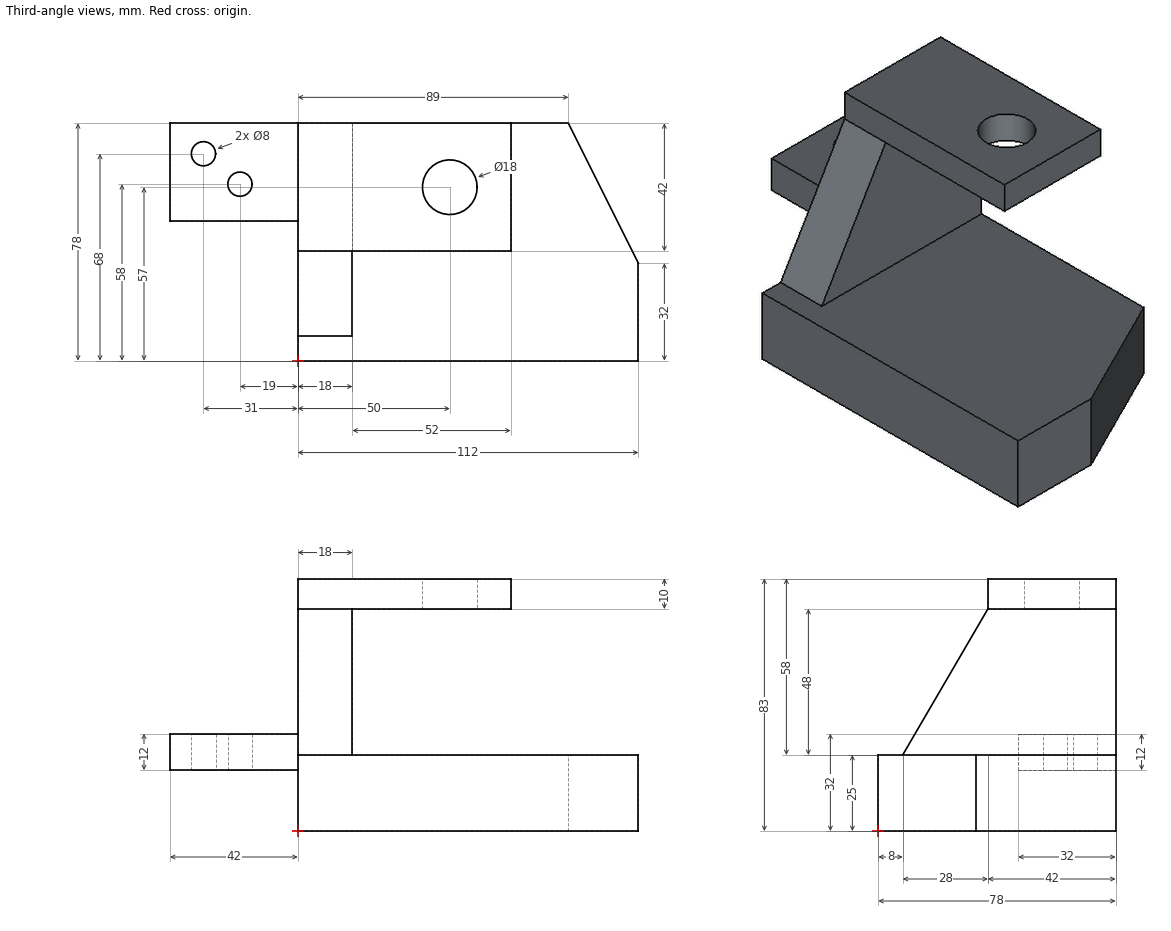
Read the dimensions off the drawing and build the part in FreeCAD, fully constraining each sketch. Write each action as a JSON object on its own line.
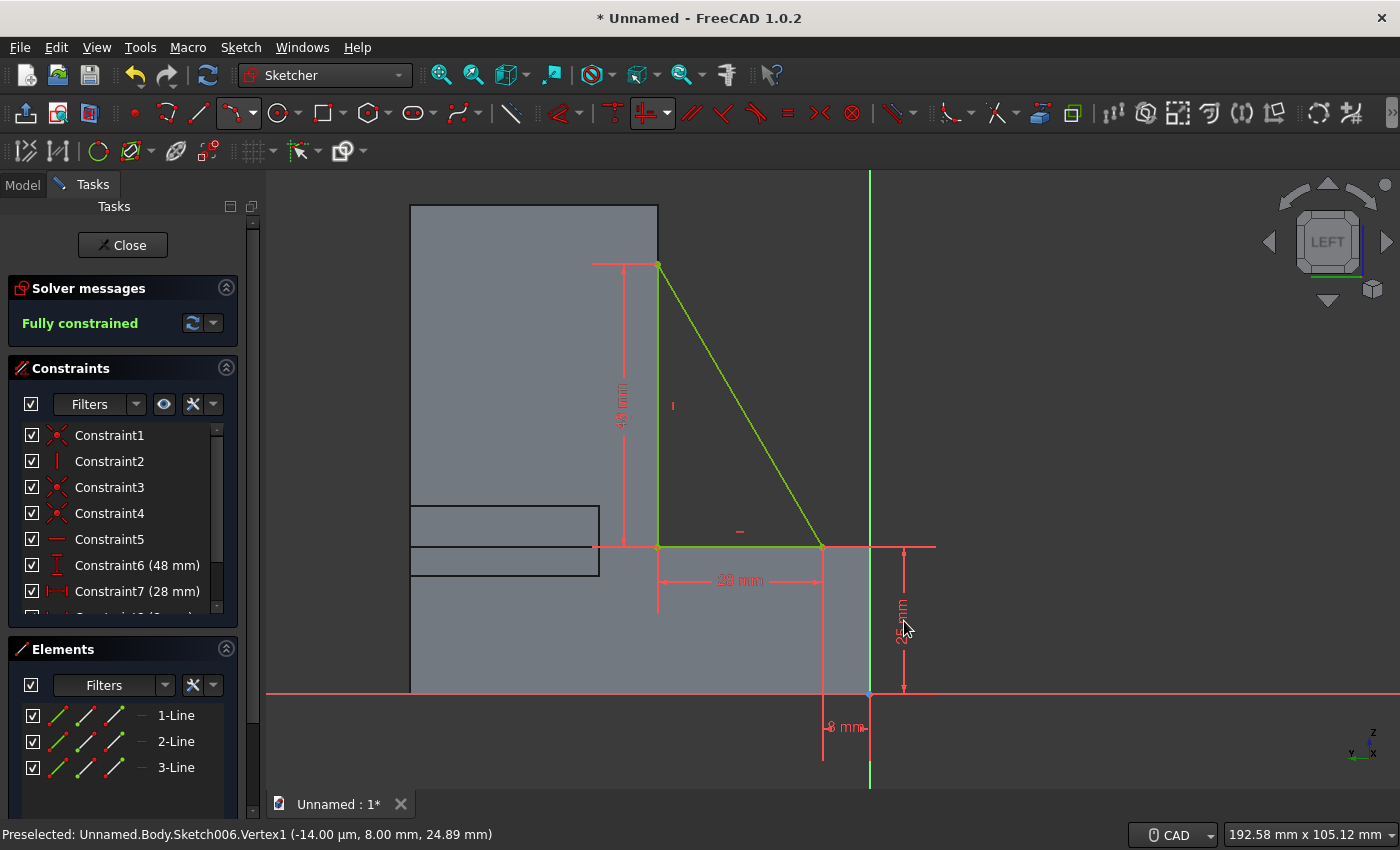
{"action": "left_click", "coordinate": [123, 245]}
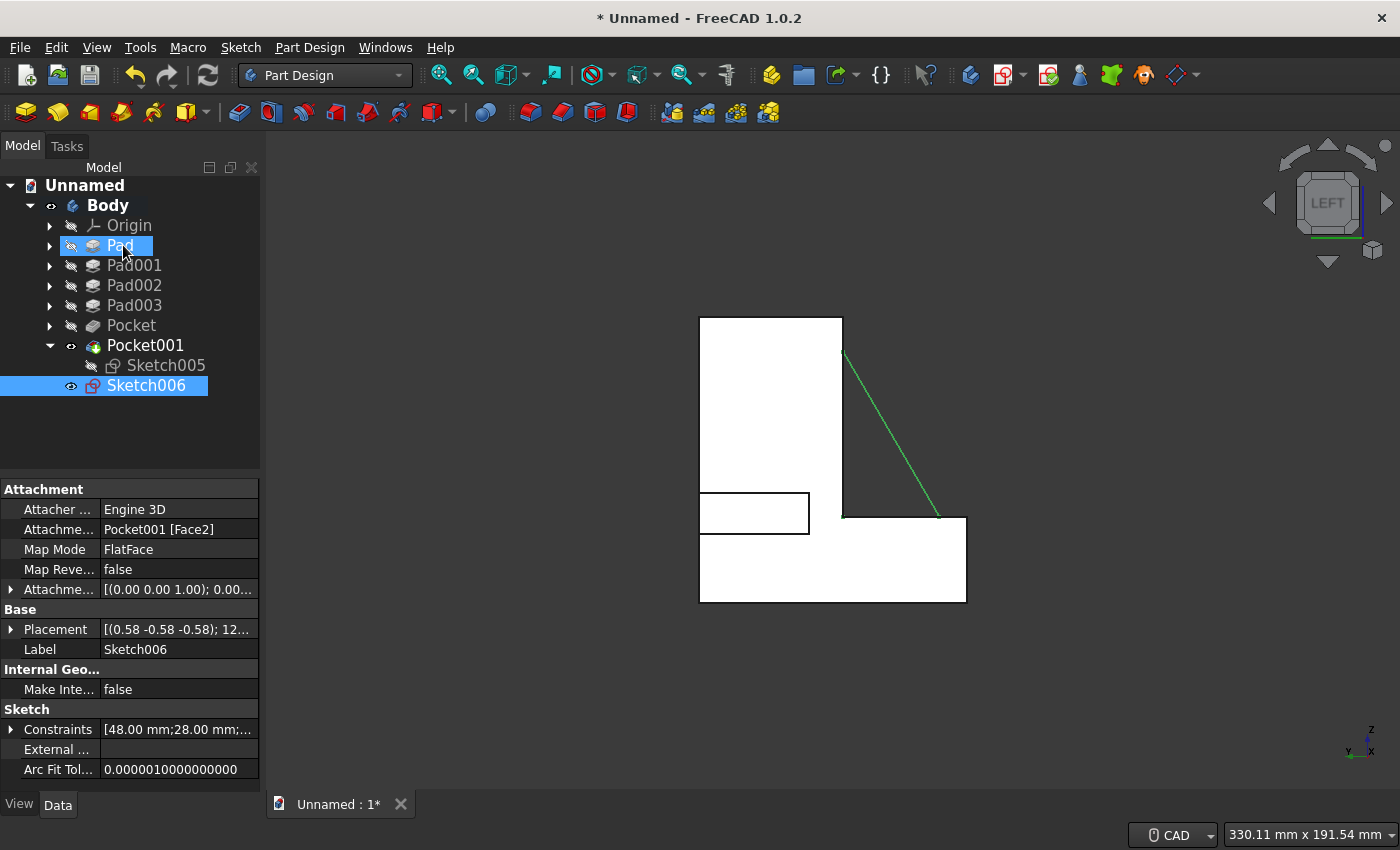
{"action": "left_click", "coordinate": [26, 112]}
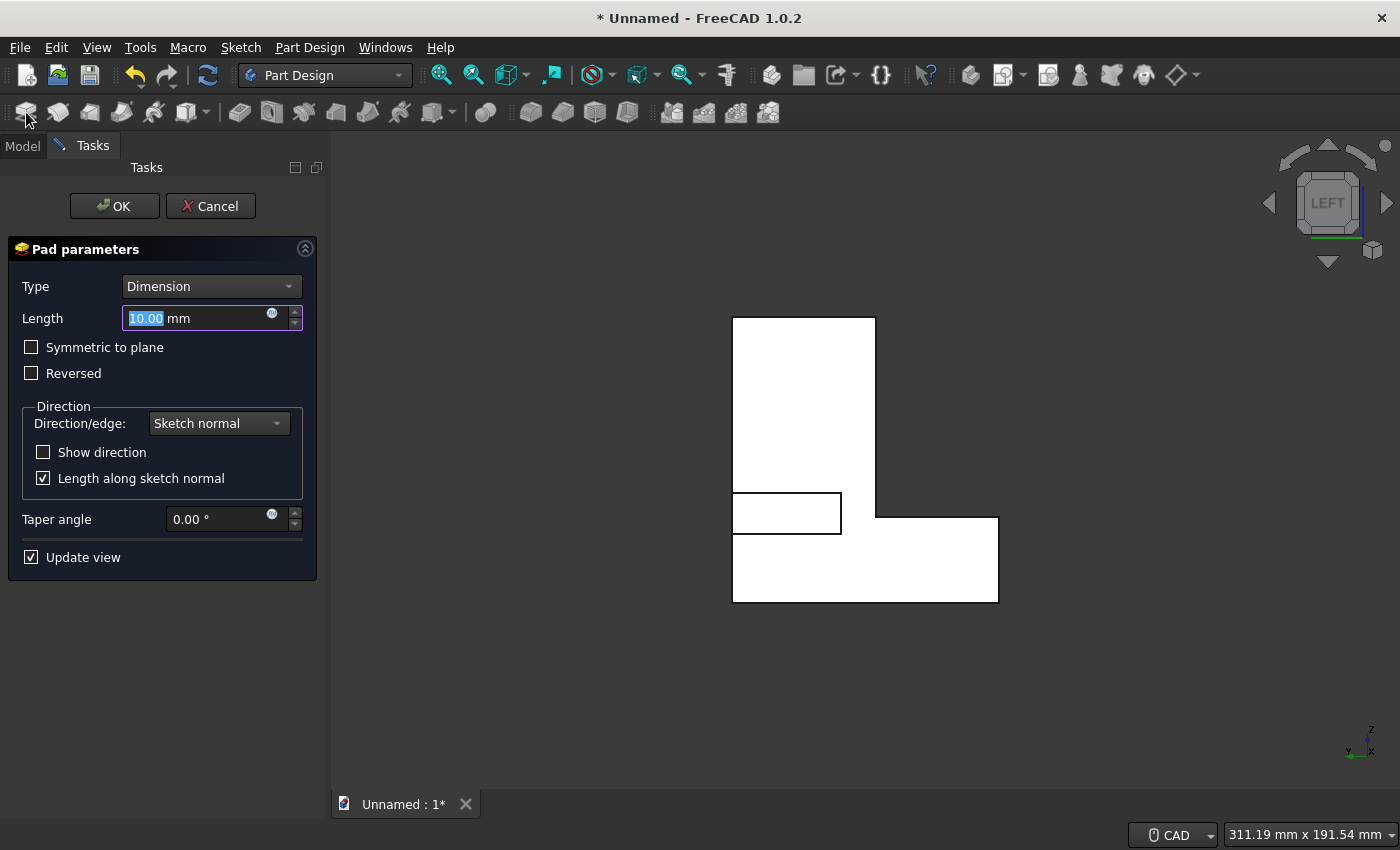
{"action": "type", "text": "18"}
{"action": "key", "text": "Tab"}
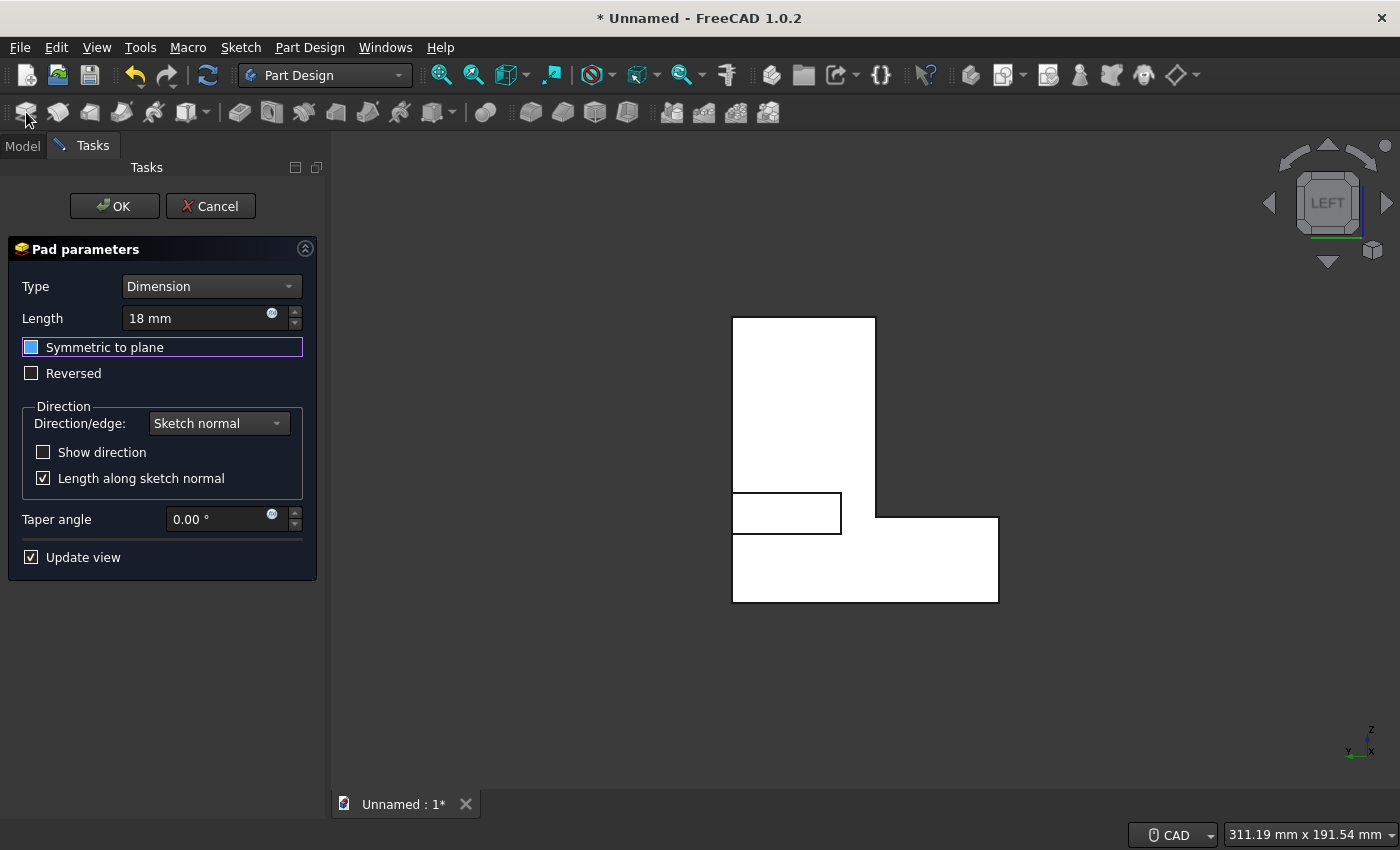
{"action": "left_click", "coordinate": [30, 373]}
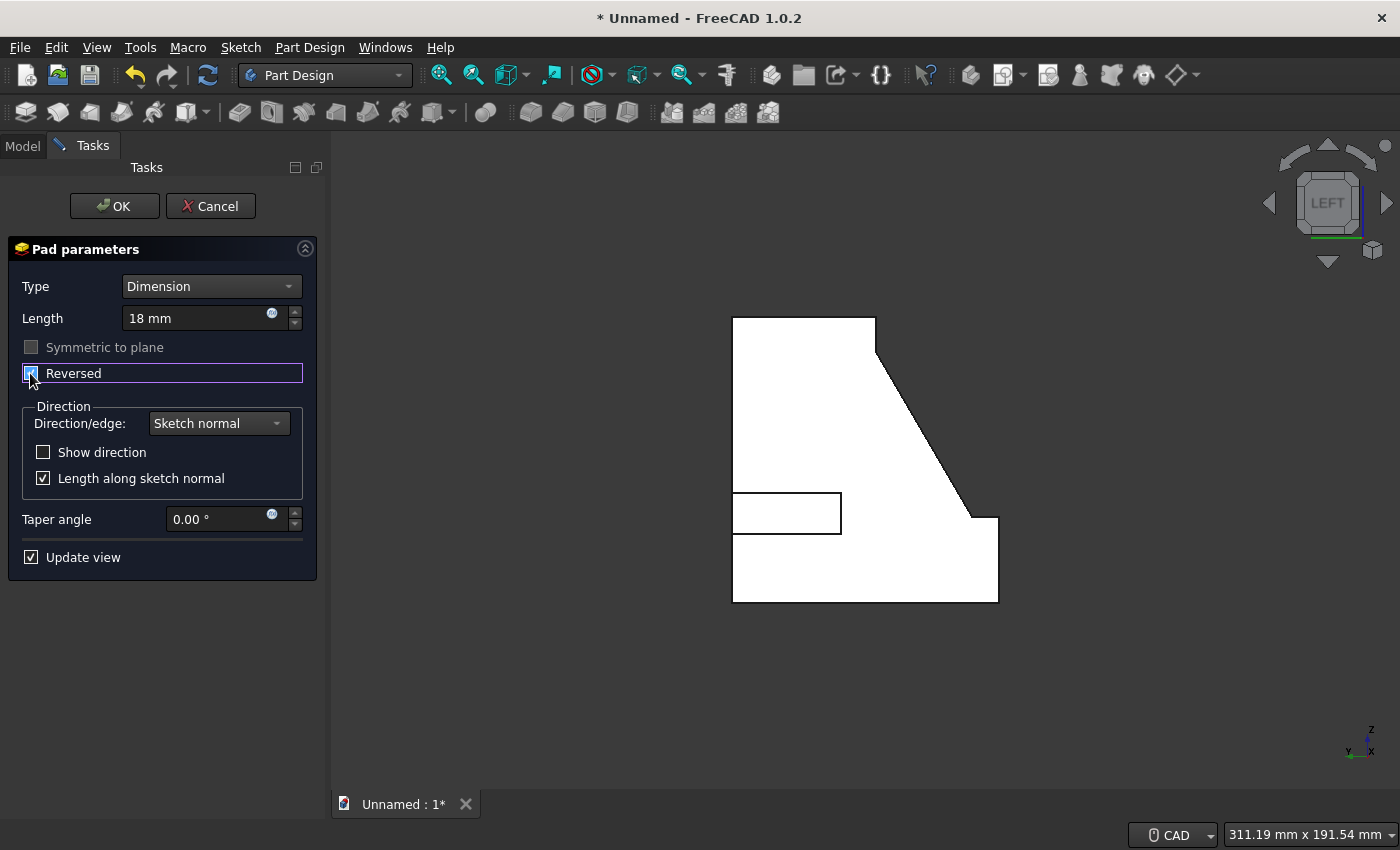
{"action": "left_click", "coordinate": [115, 206]}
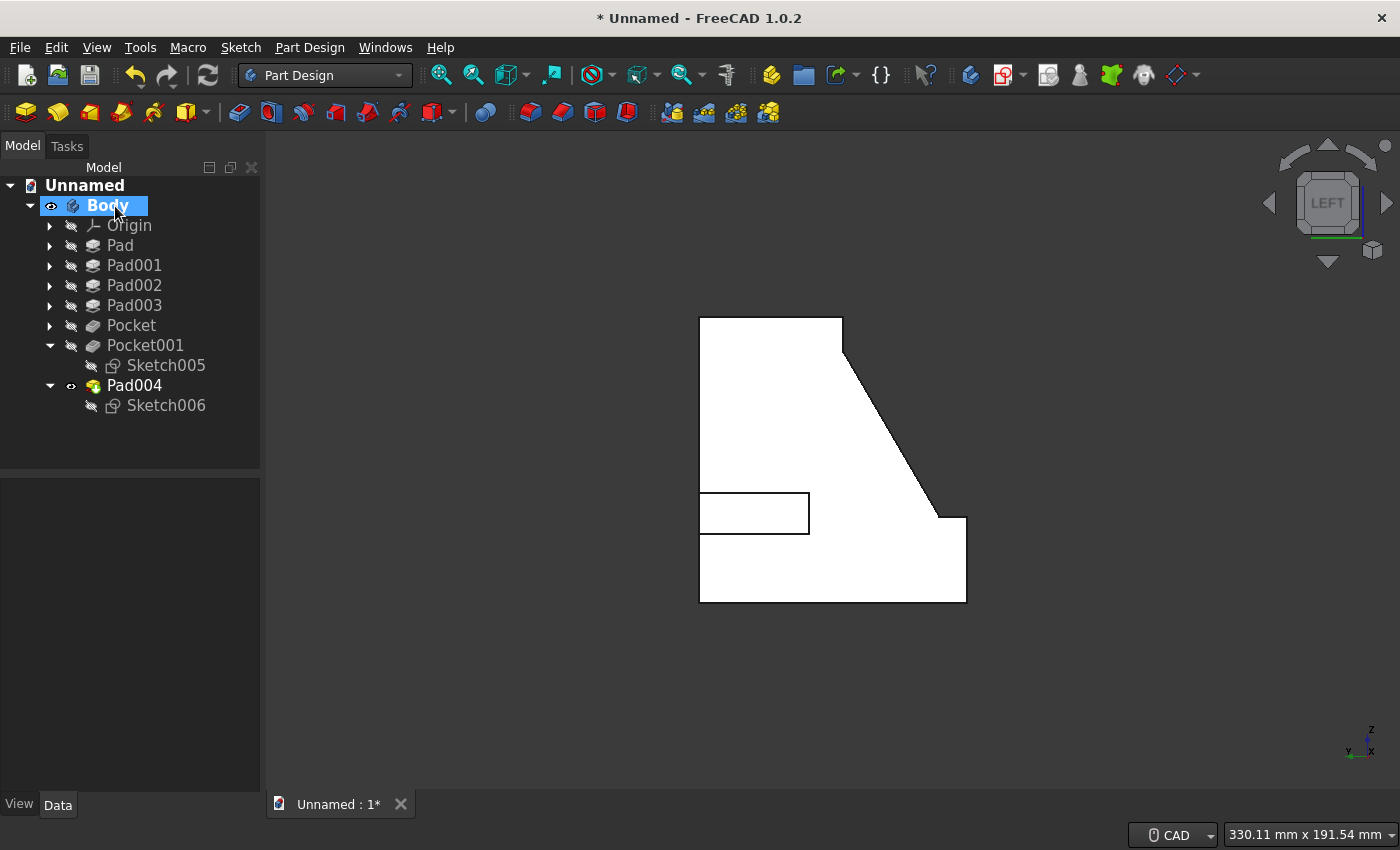
{"action": "key", "text": "0"}